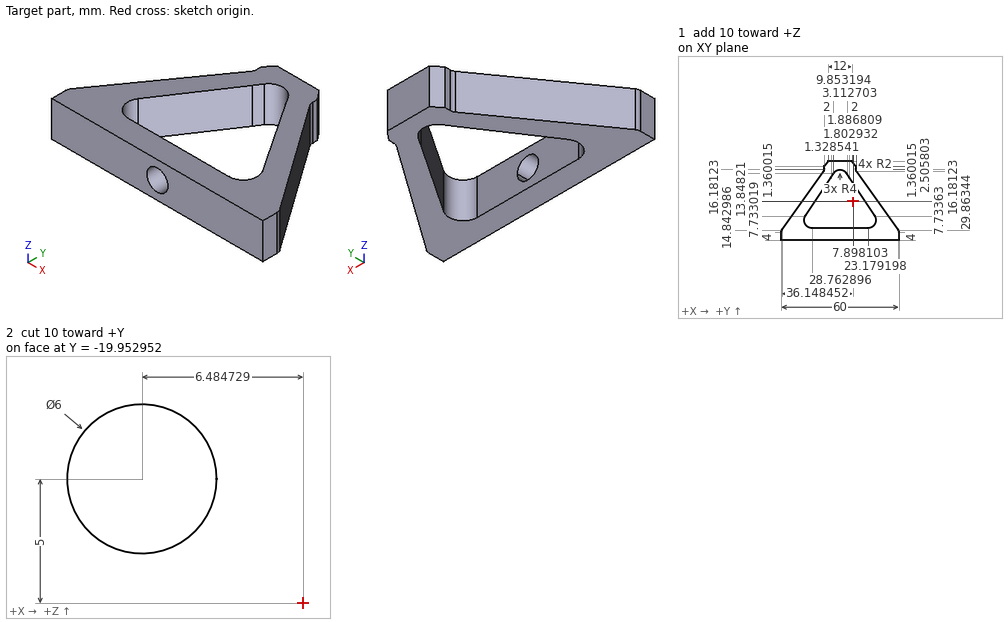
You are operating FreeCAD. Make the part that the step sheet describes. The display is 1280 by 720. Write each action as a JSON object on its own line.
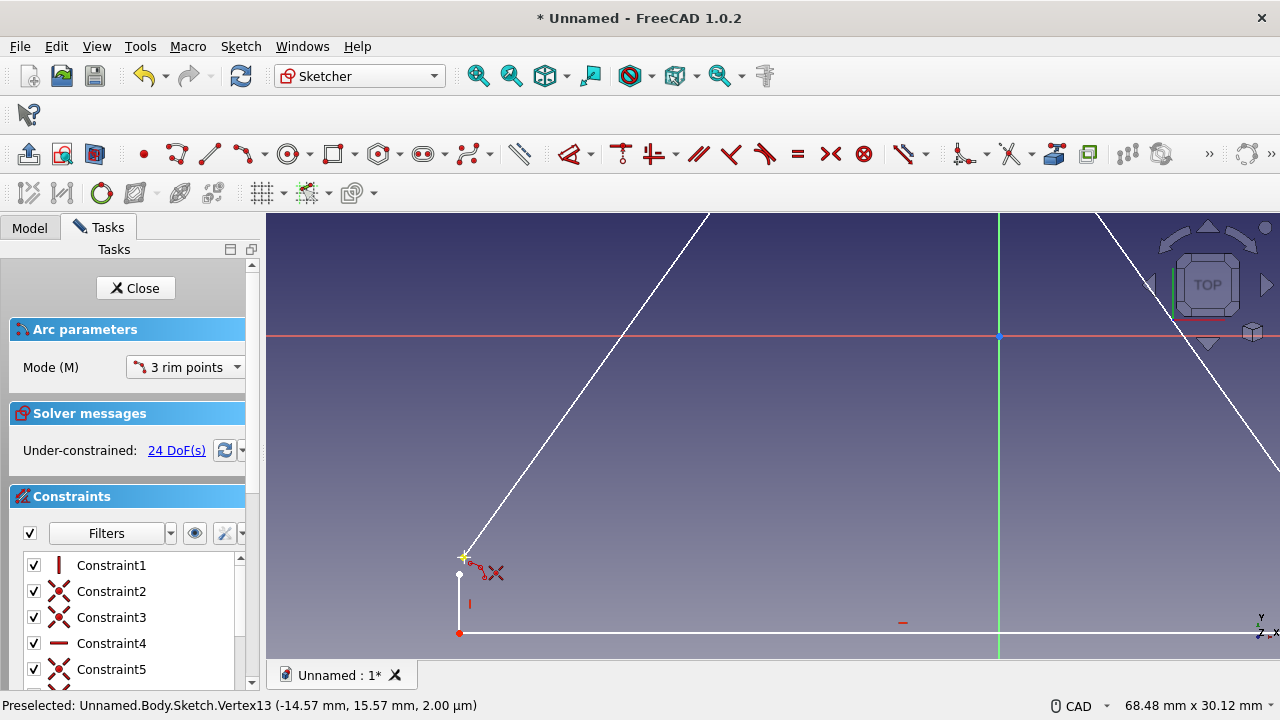
{"action": "left_click", "coordinate": [463, 558]}
{"action": "left_click", "coordinate": [459, 574]}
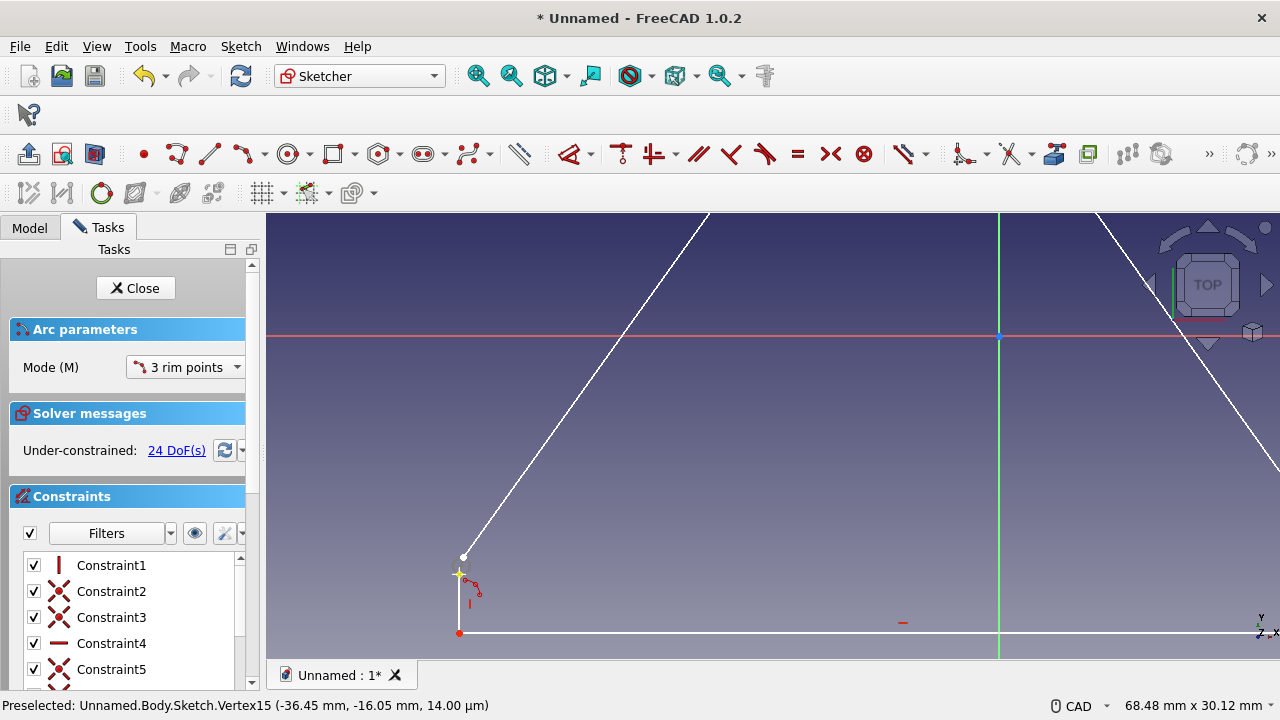
{"action": "scroll", "coordinate": [460, 564], "scroll_direction": "up", "scroll_amount": 13}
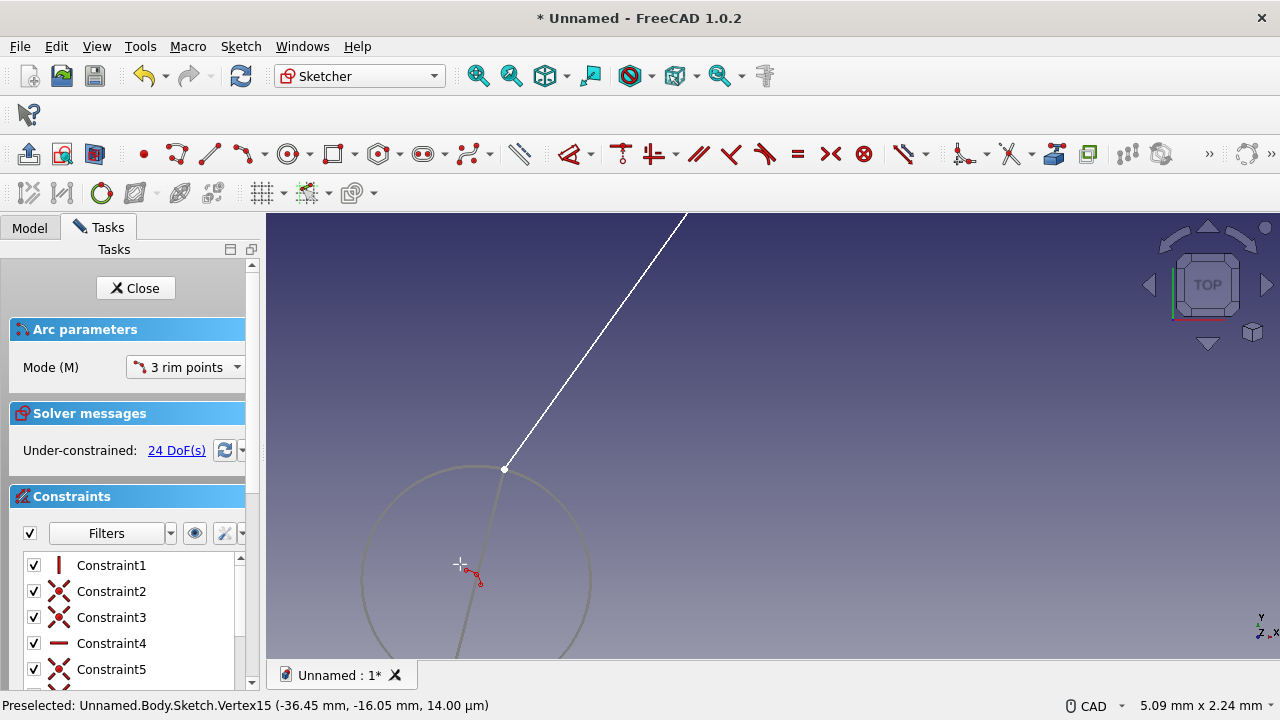
{"action": "left_click", "coordinate": [459, 556]}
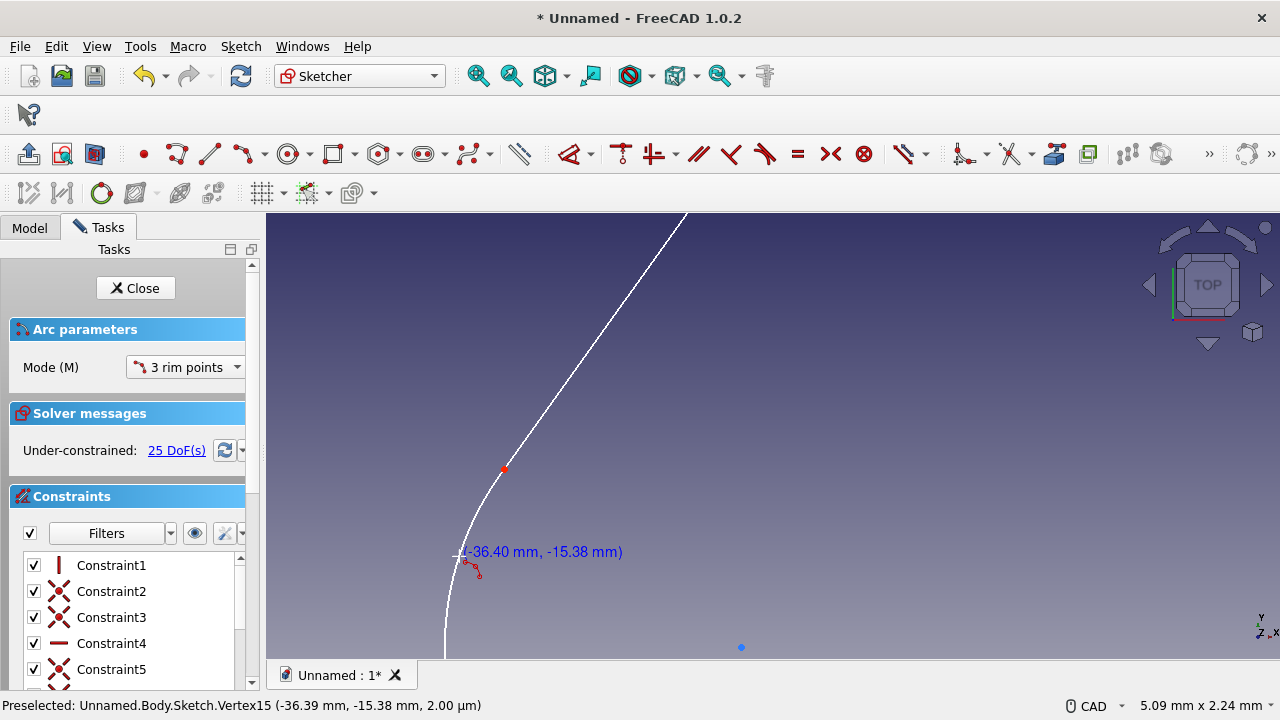
{"action": "scroll", "coordinate": [462, 562], "scroll_direction": "down", "scroll_amount": 16}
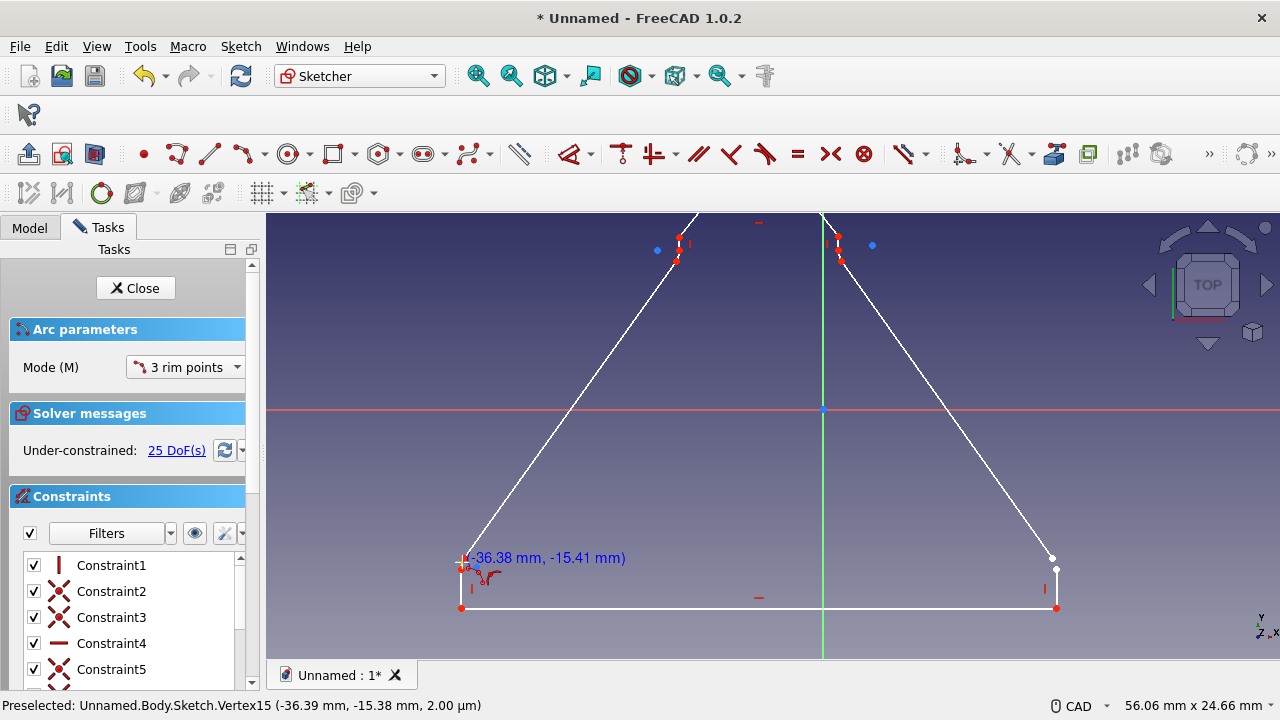
{"action": "scroll", "coordinate": [949, 567], "scroll_direction": "up", "scroll_amount": 3}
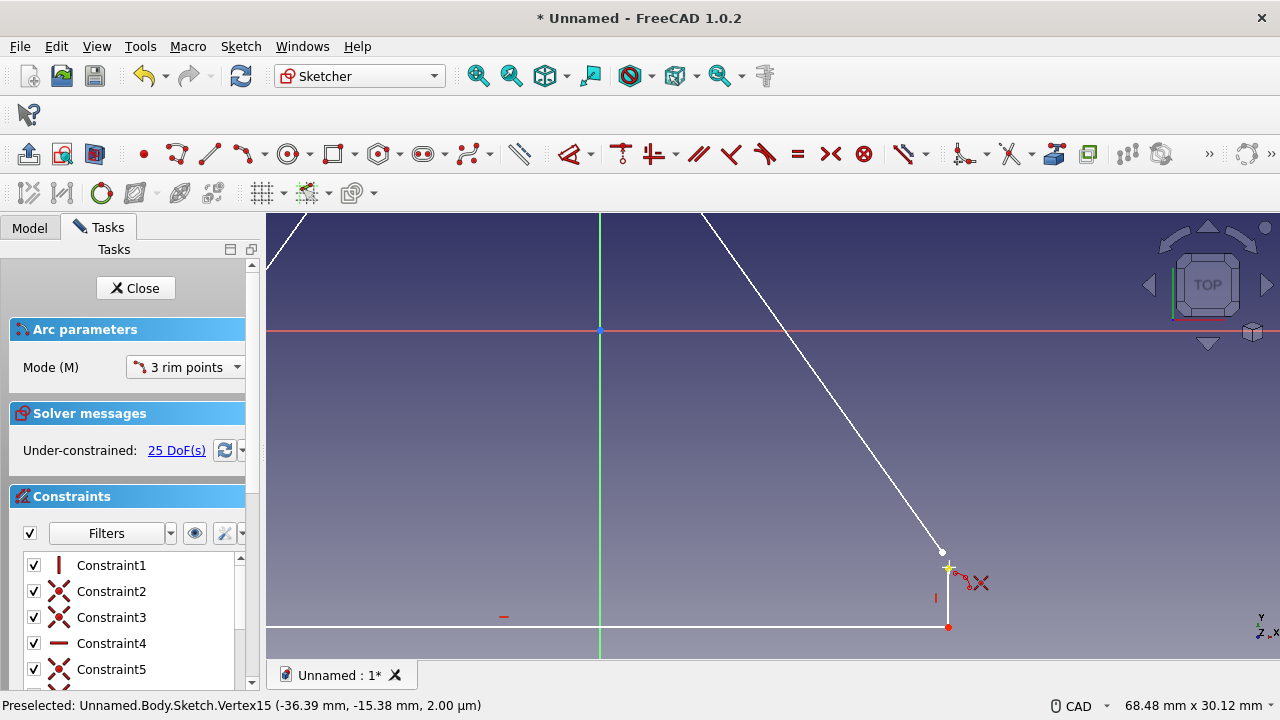
{"action": "left_click", "coordinate": [948, 568]}
{"action": "left_click", "coordinate": [943, 553]}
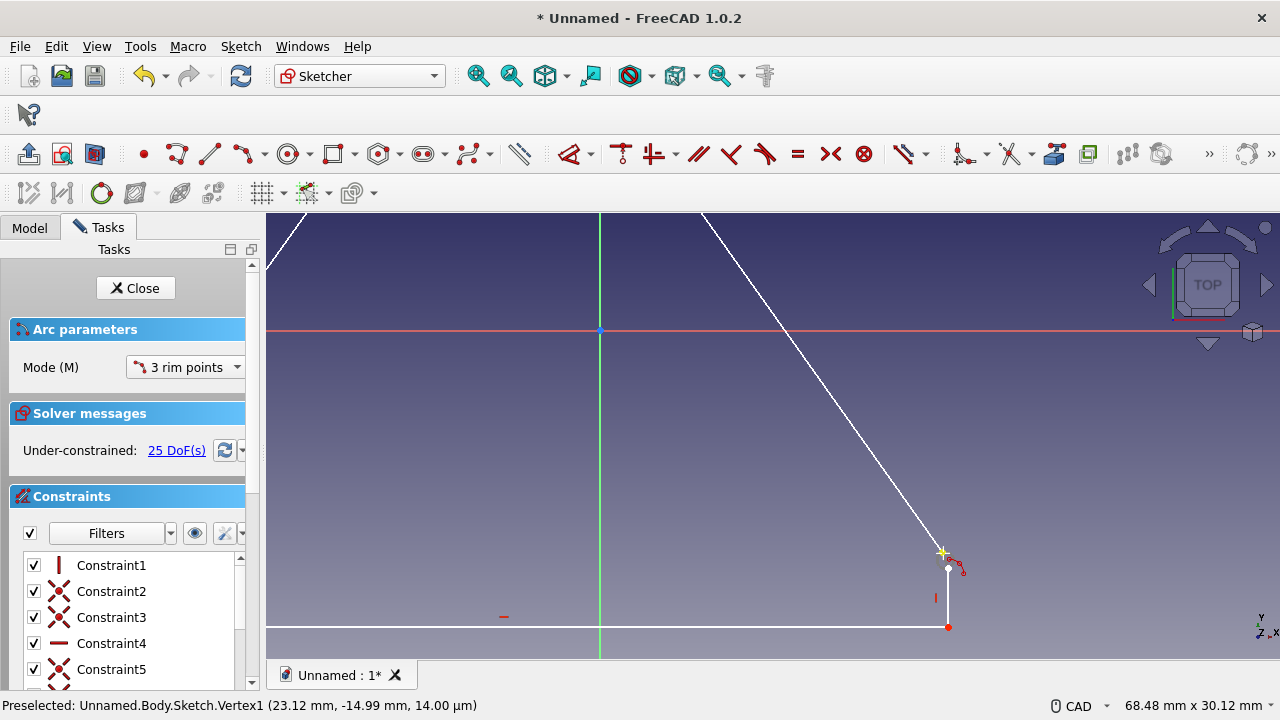
{"action": "scroll", "coordinate": [947, 558], "scroll_direction": "up", "scroll_amount": 13}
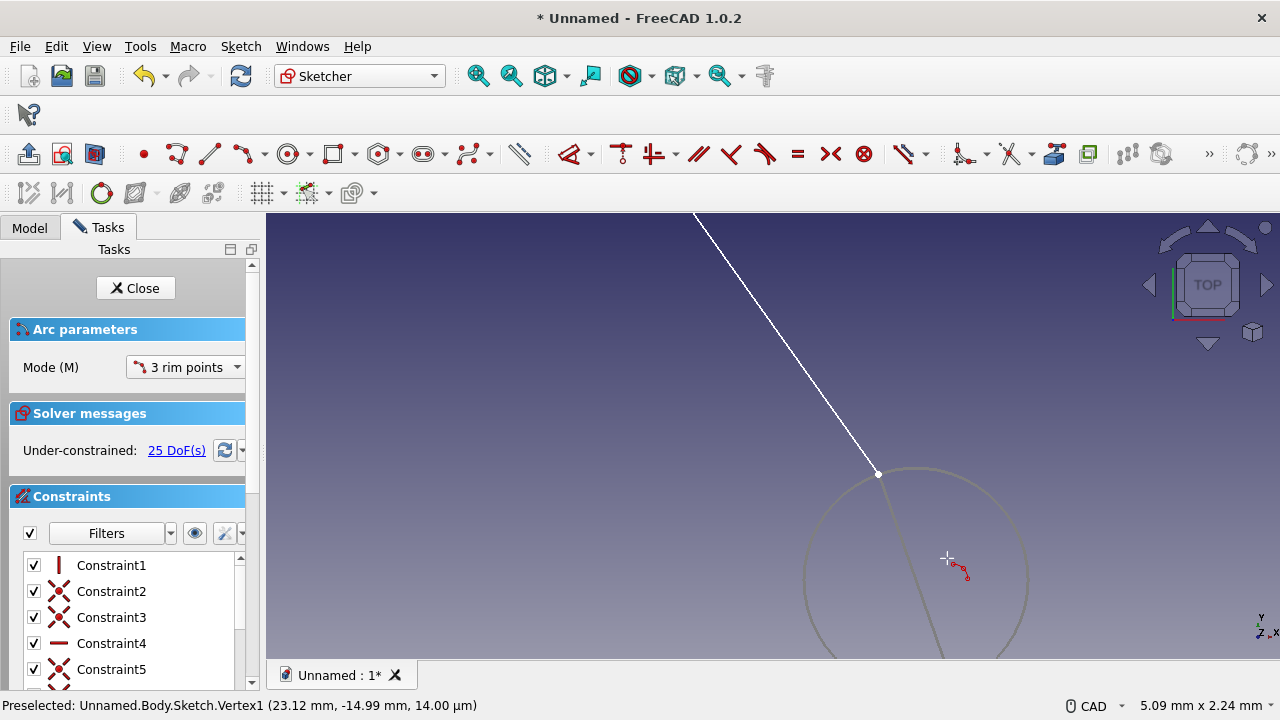
{"action": "left_click", "coordinate": [940, 550]}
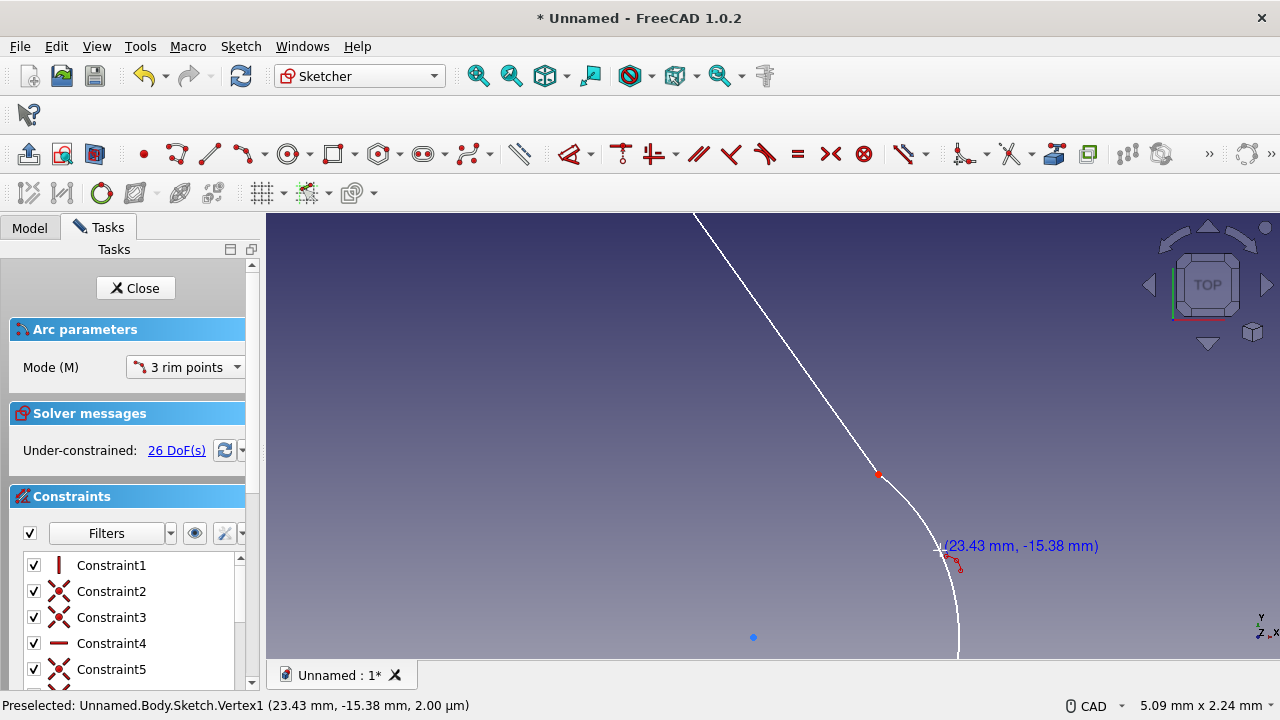
{"action": "left_click", "coordinate": [177, 154]}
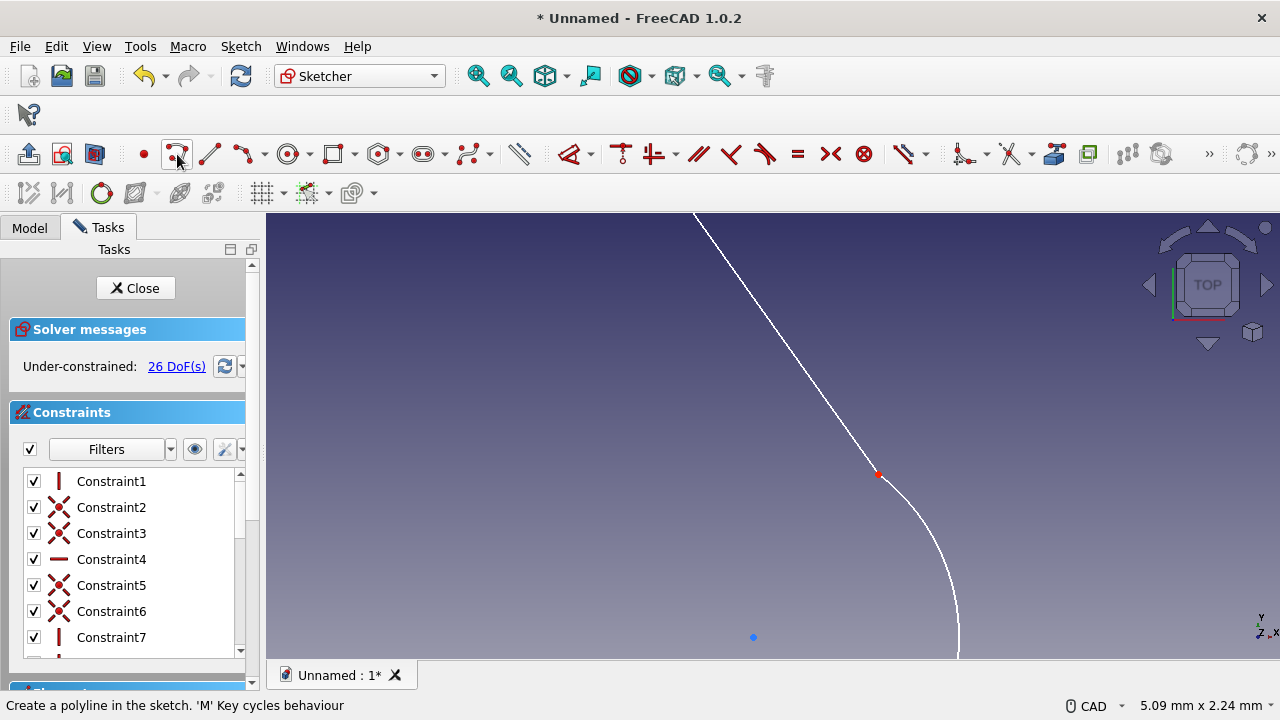
{"action": "scroll", "coordinate": [948, 562], "scroll_direction": "down", "scroll_amount": 16}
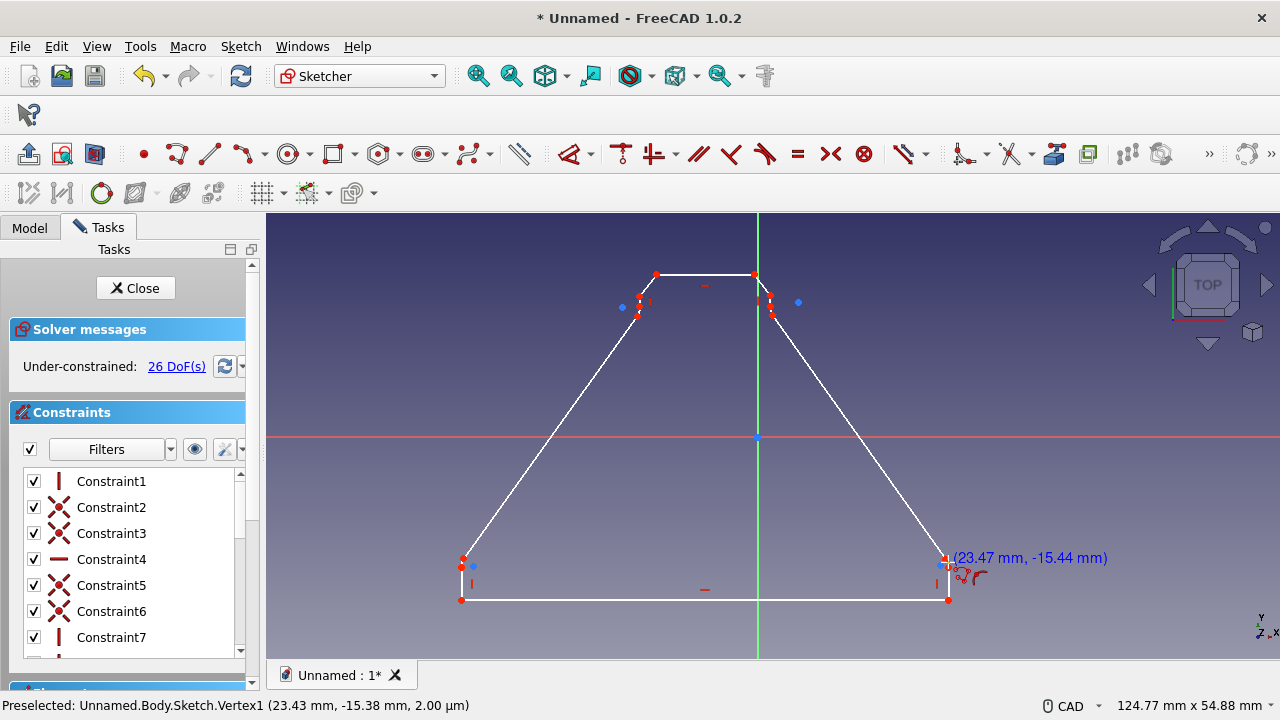
{"action": "left_click", "coordinate": [561, 500]}
{"action": "left_click", "coordinate": [667, 342]}
{"action": "left_click", "coordinate": [678, 325]}
{"action": "right_click", "coordinate": [678, 325]}